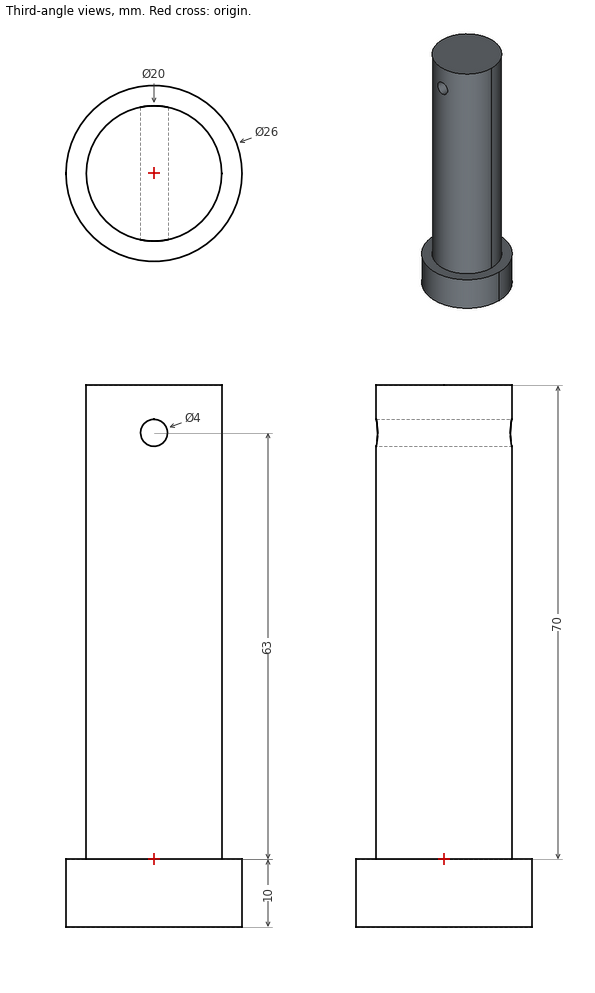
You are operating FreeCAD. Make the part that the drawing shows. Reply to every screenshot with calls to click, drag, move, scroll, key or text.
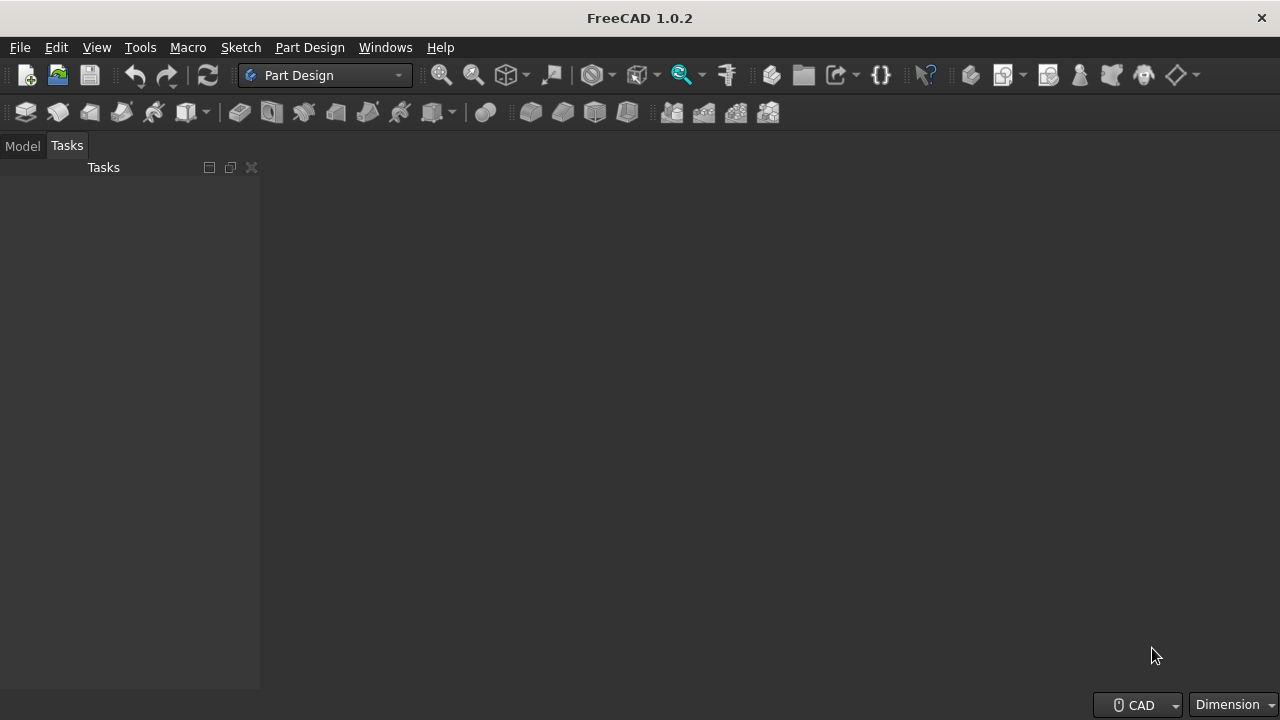
click(26, 76)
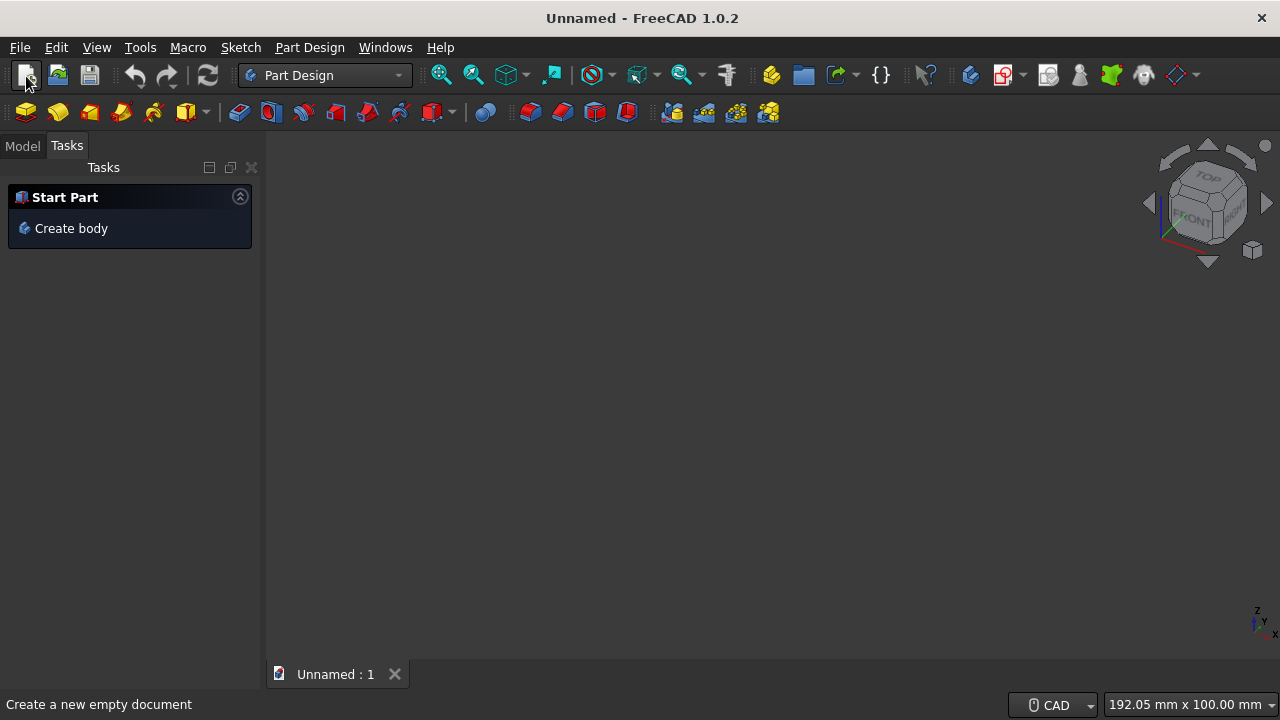
click(1004, 76)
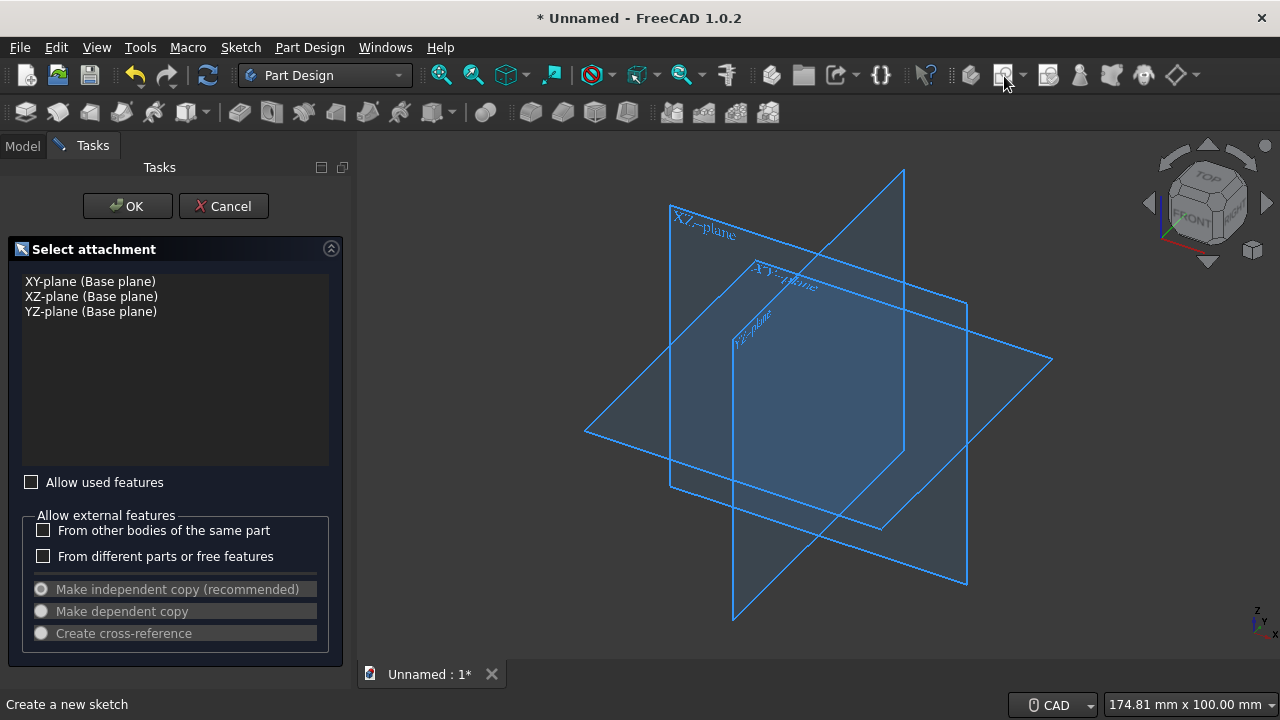
click(82, 282)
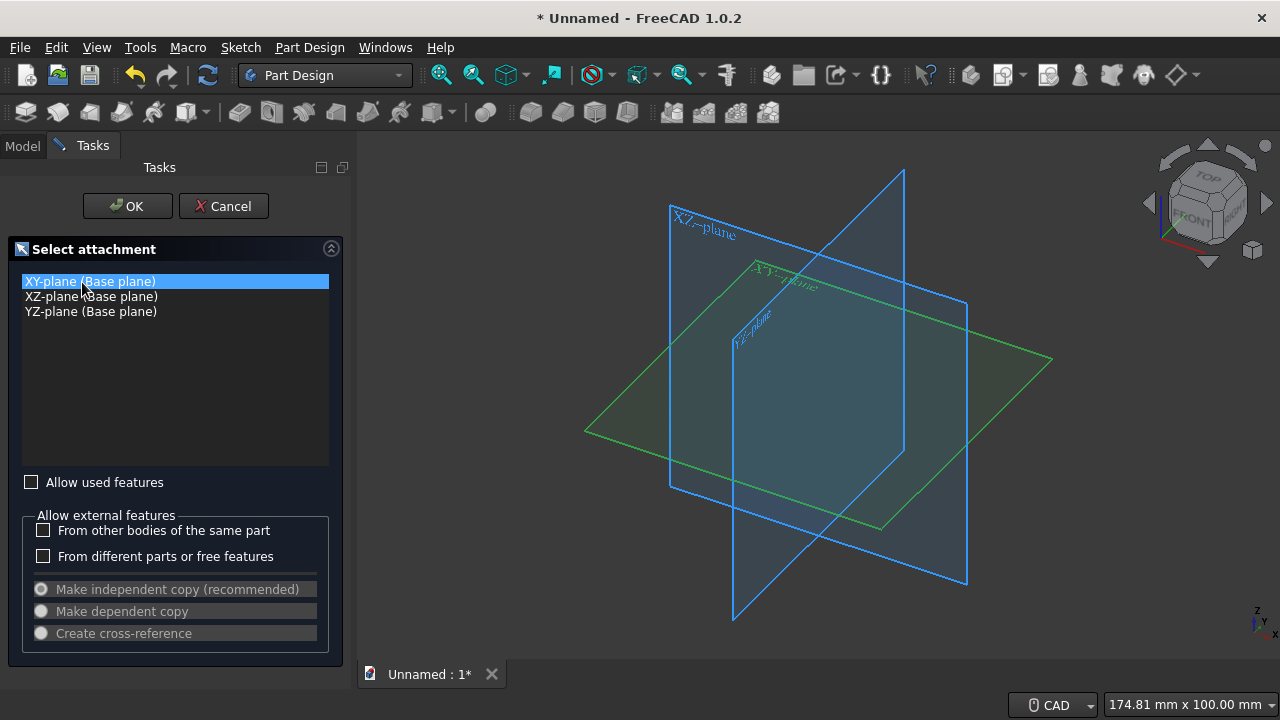
click(128, 206)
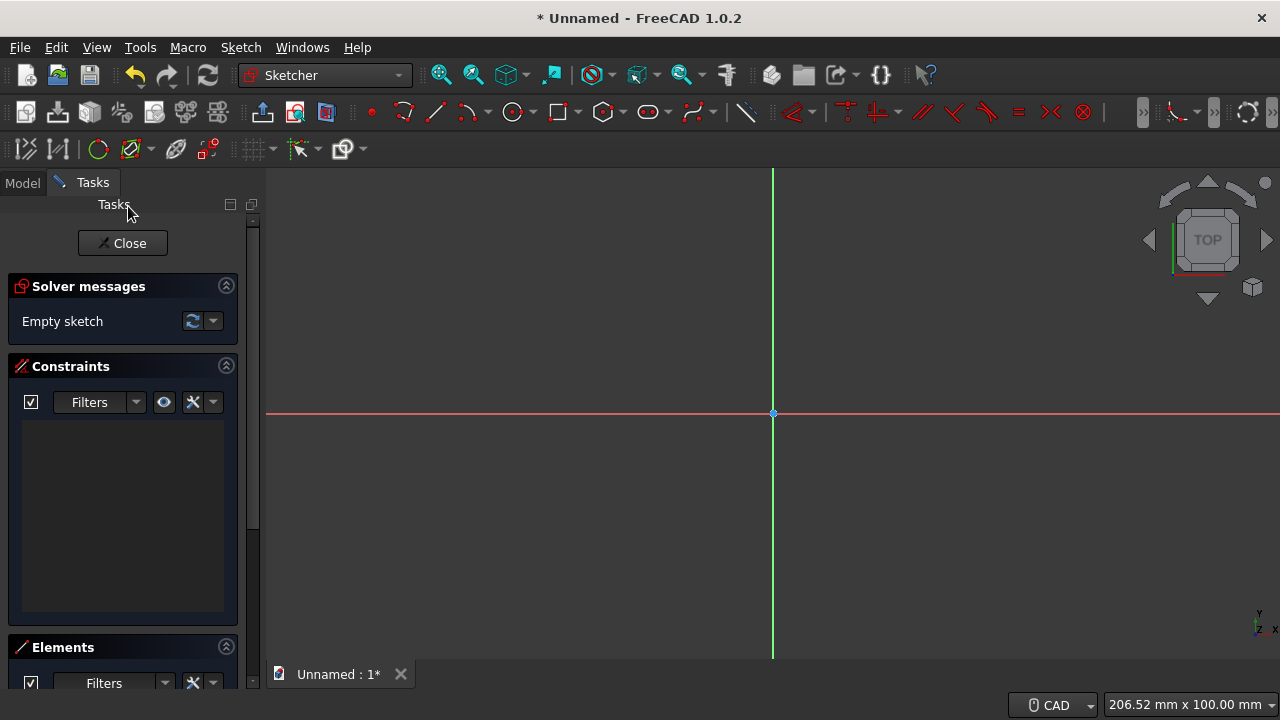
scroll(803, 414, up, 6)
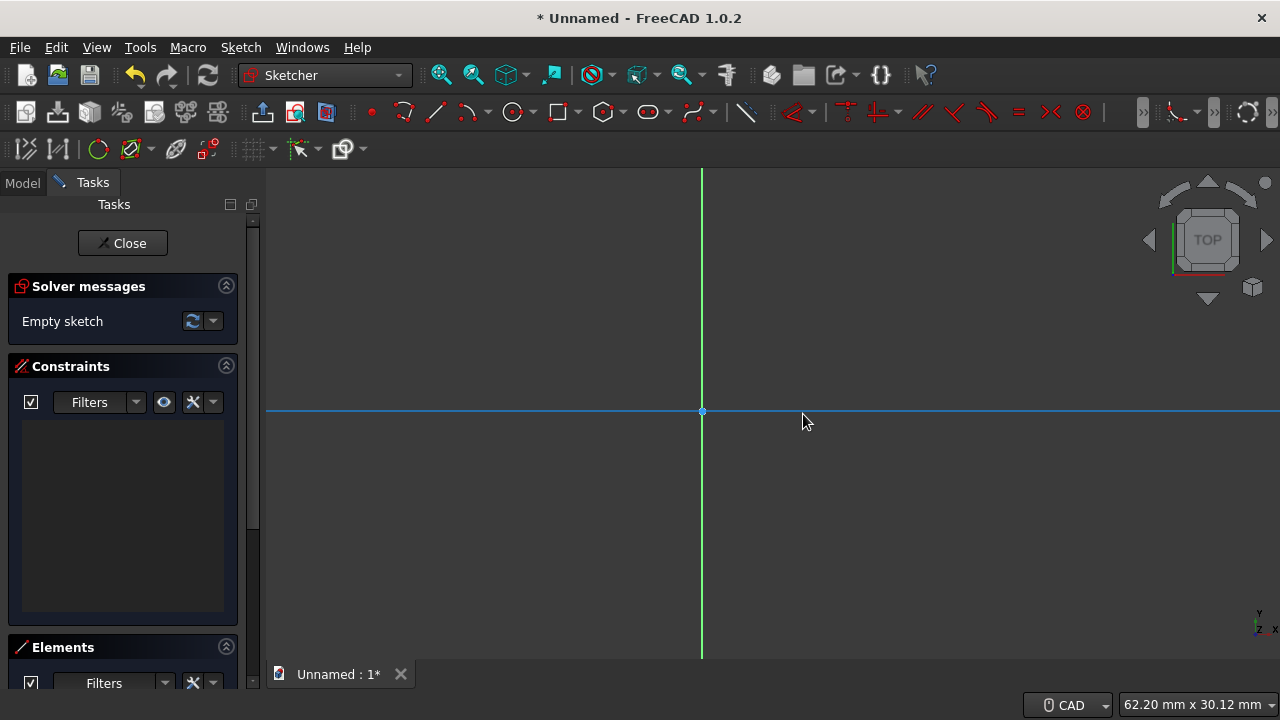
click(514, 112)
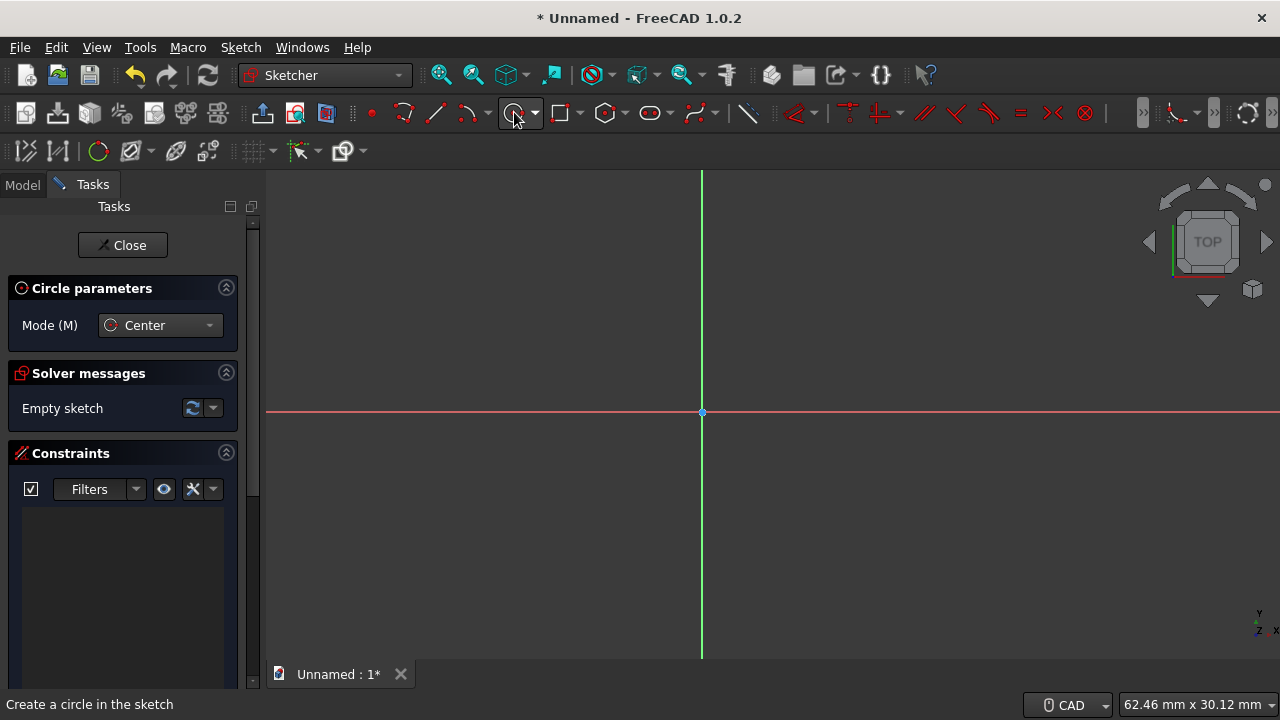
click(702, 412)
move(817, 297)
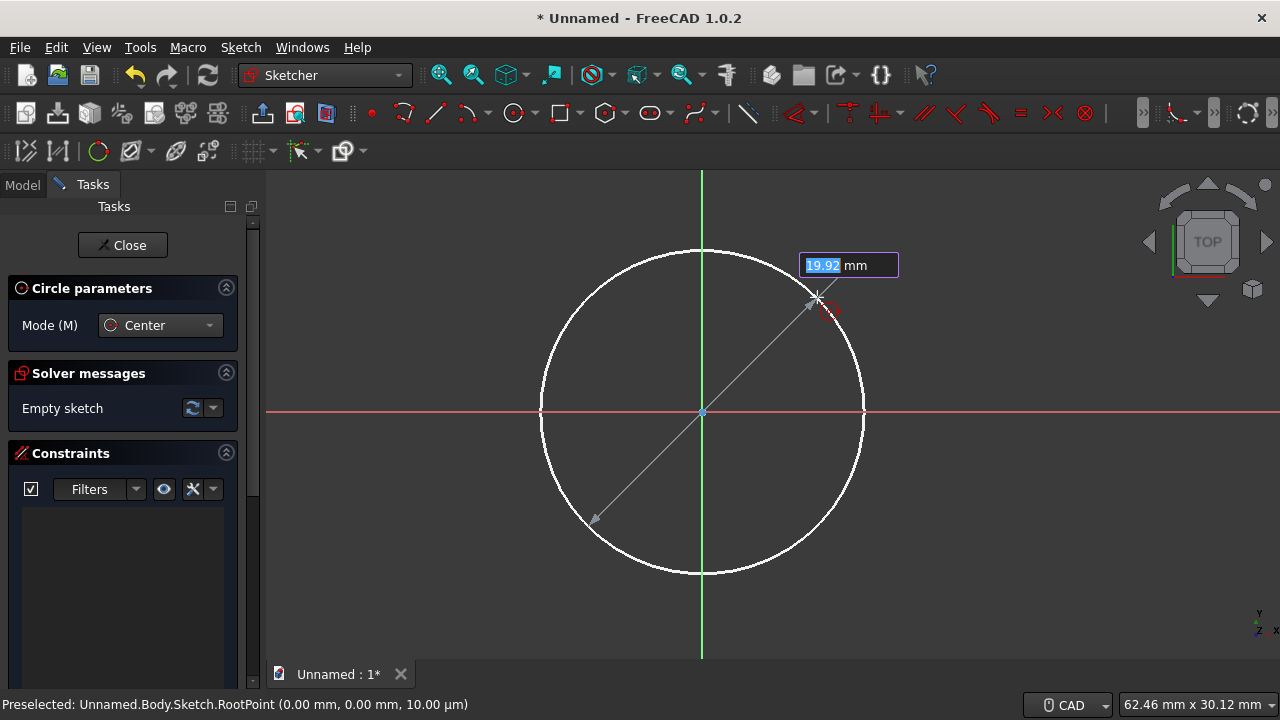
text(20)
key(Return)
key(Escape)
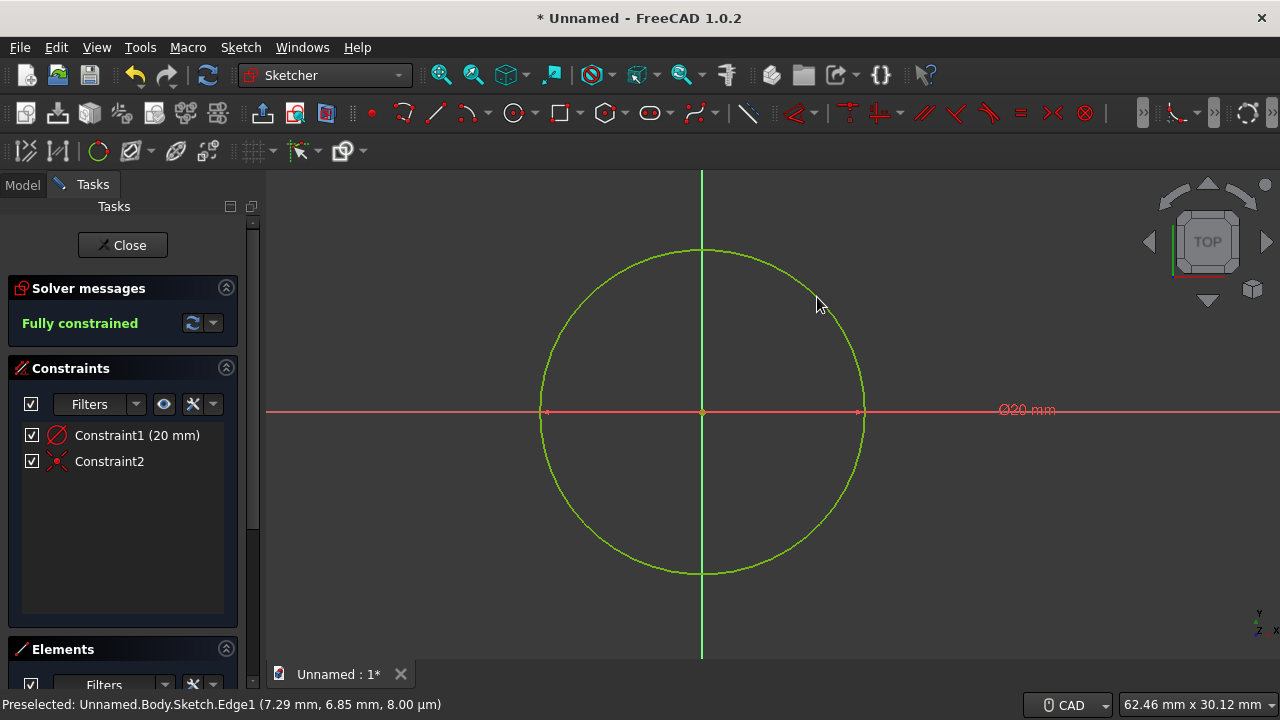
click(123, 245)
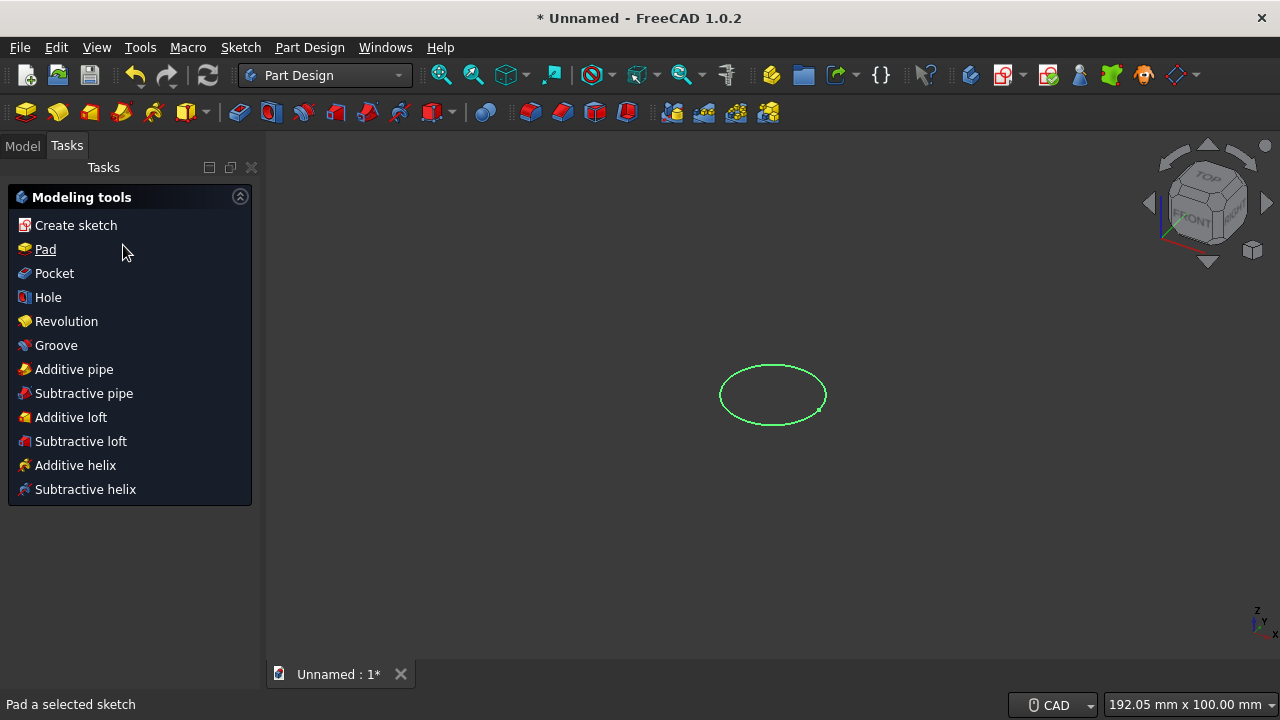
click(26, 112)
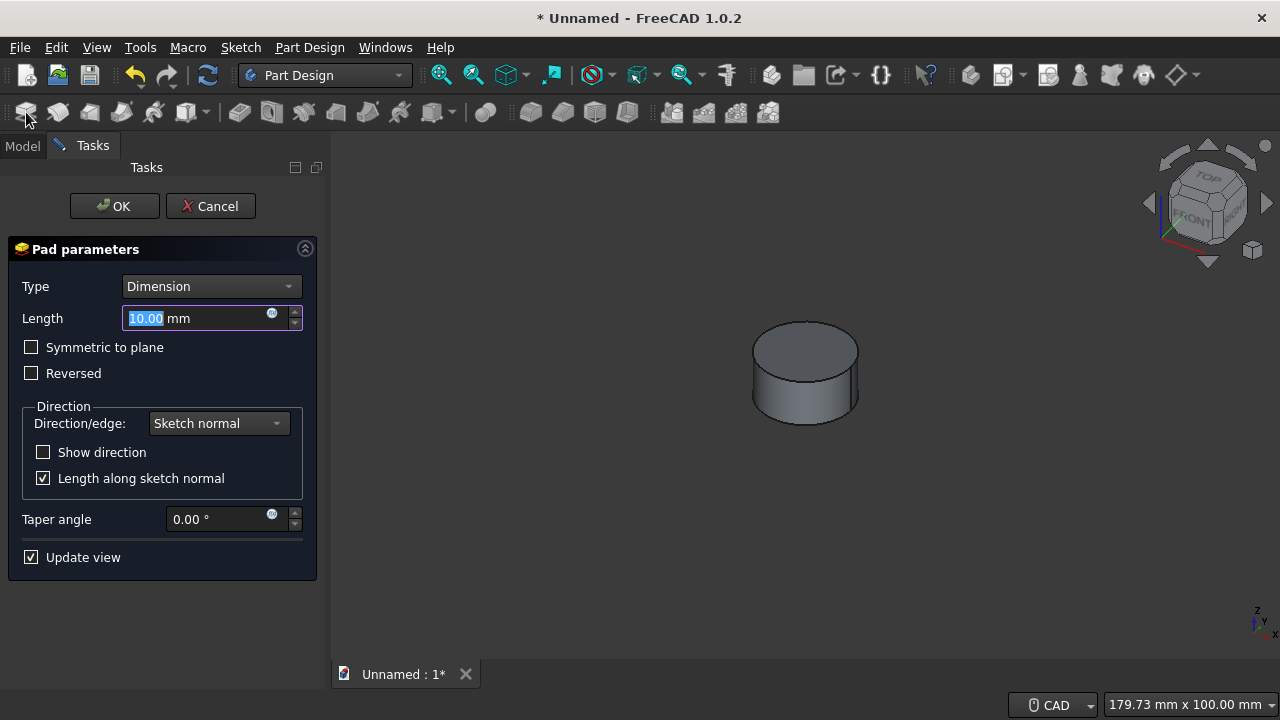
text(70)
key(Tab)